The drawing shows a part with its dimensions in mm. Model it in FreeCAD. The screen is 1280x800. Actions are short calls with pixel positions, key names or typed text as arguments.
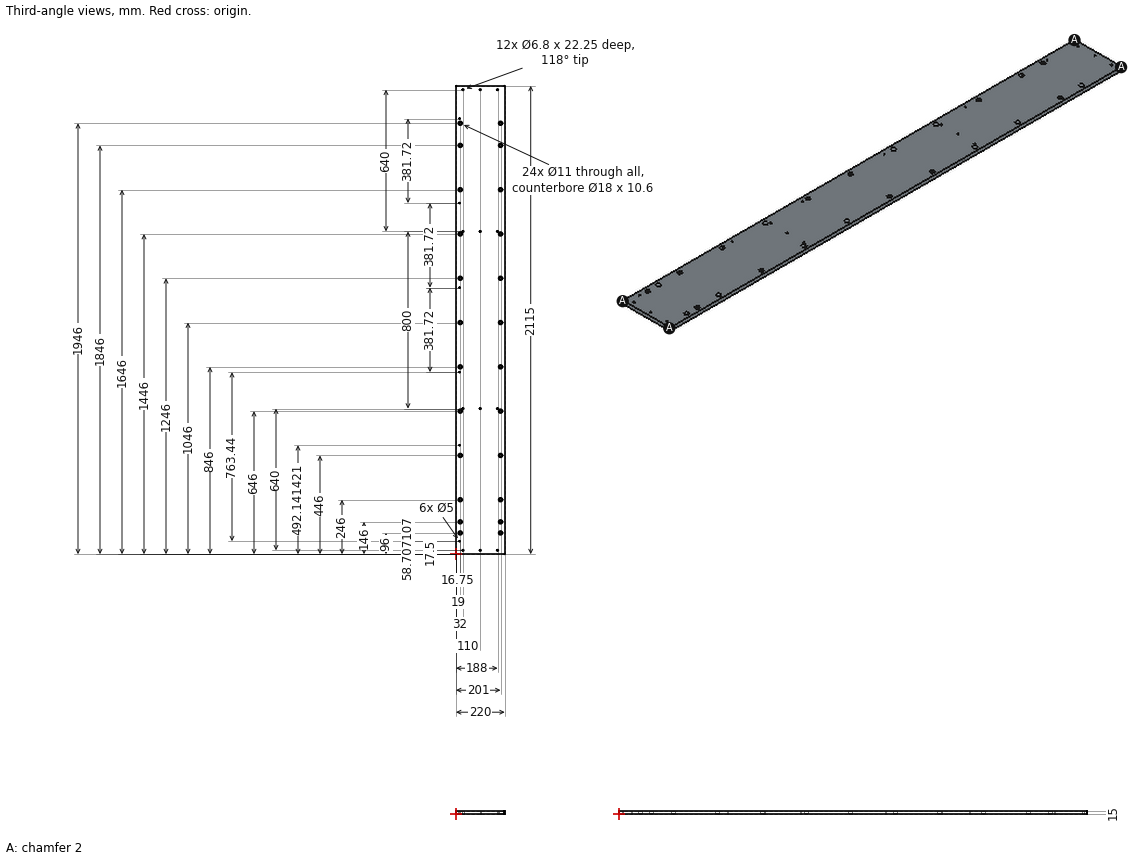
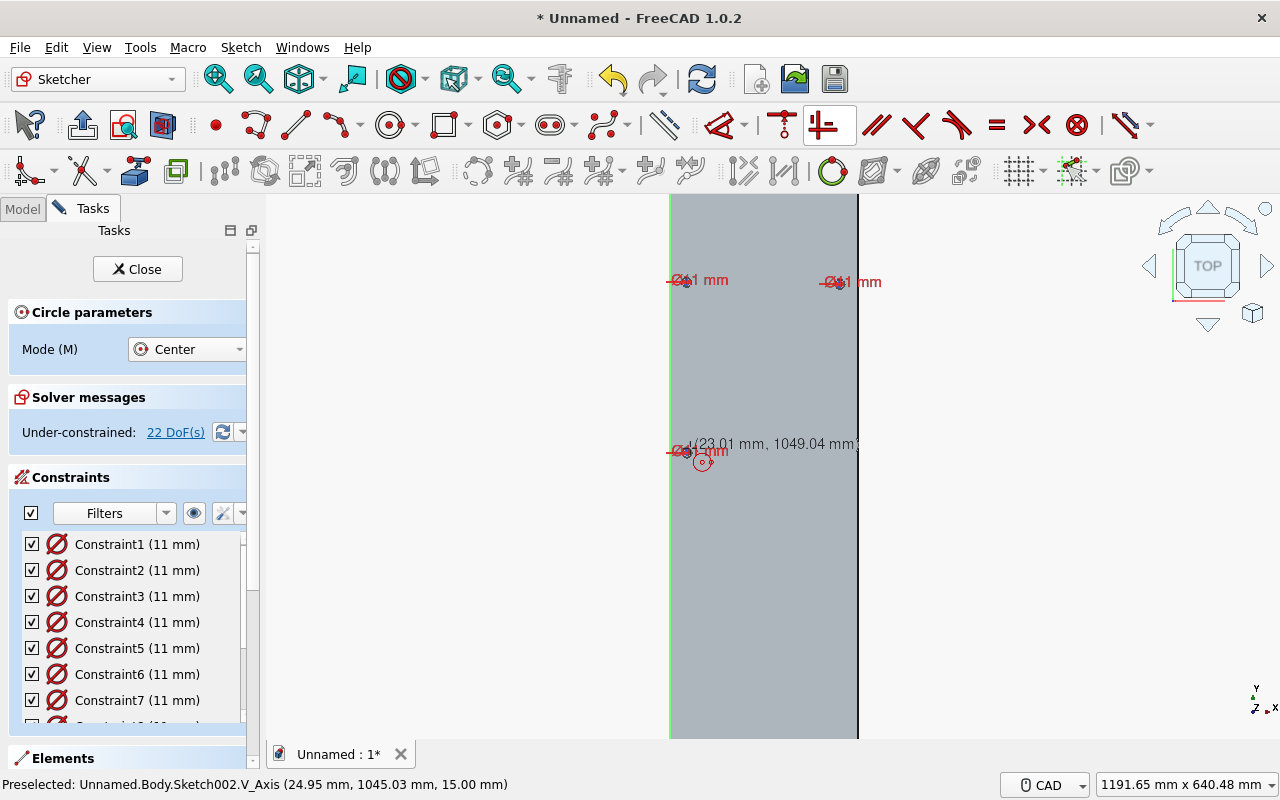
scroll(841, 452, up, 8)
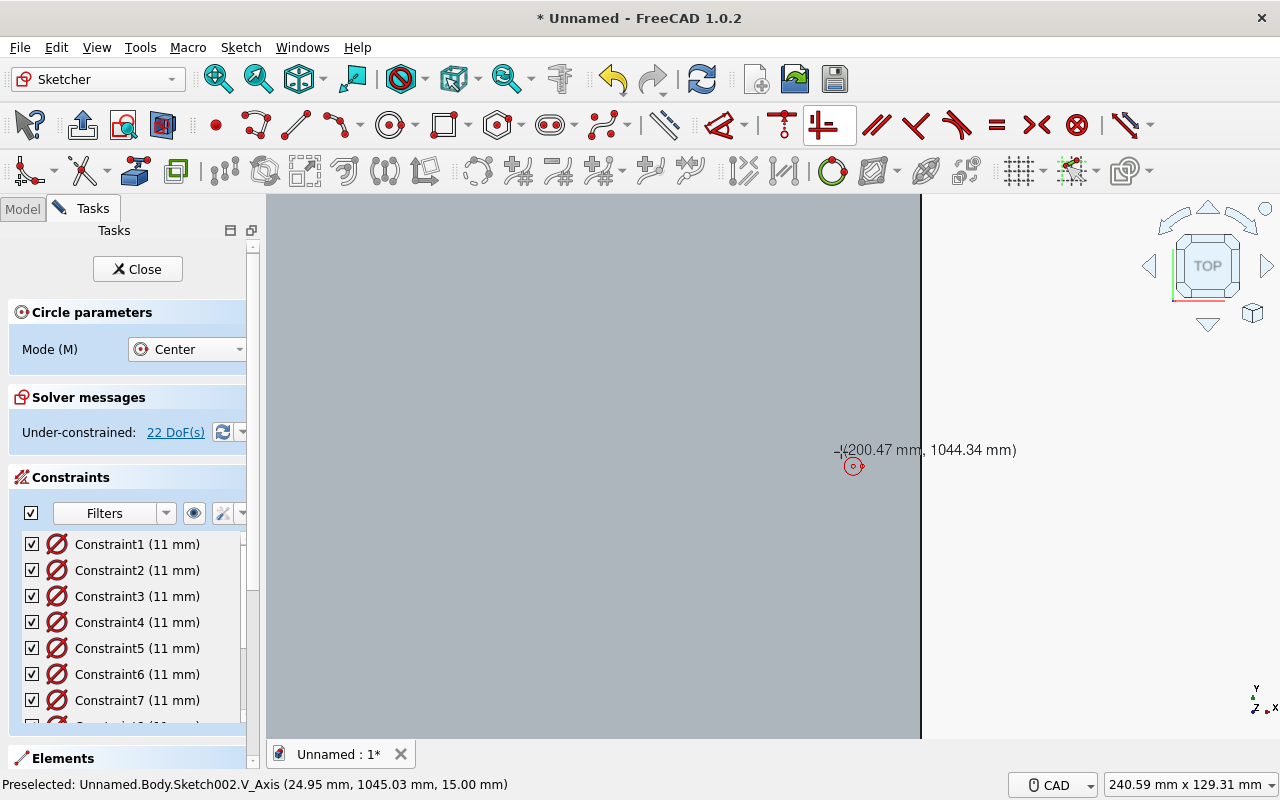
scroll(719, 452, down, 15)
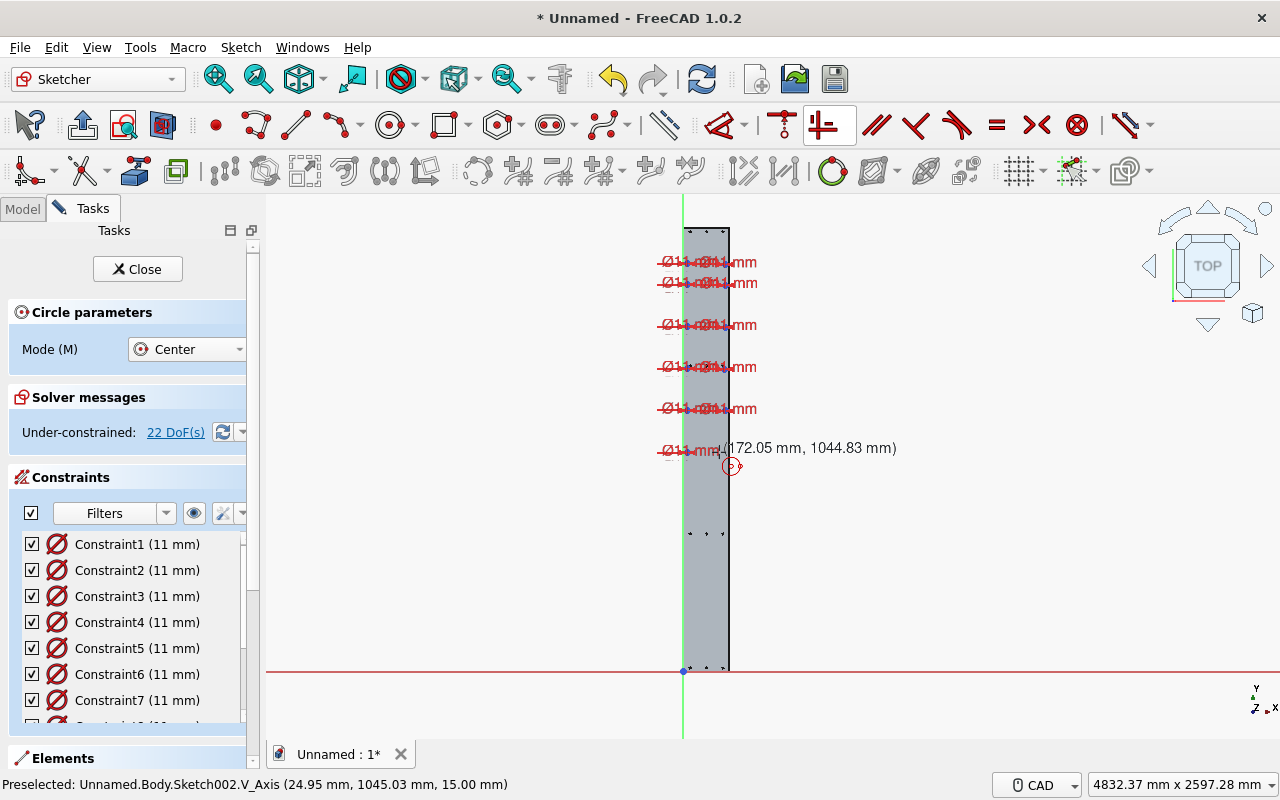
click(725, 452)
move(726, 451)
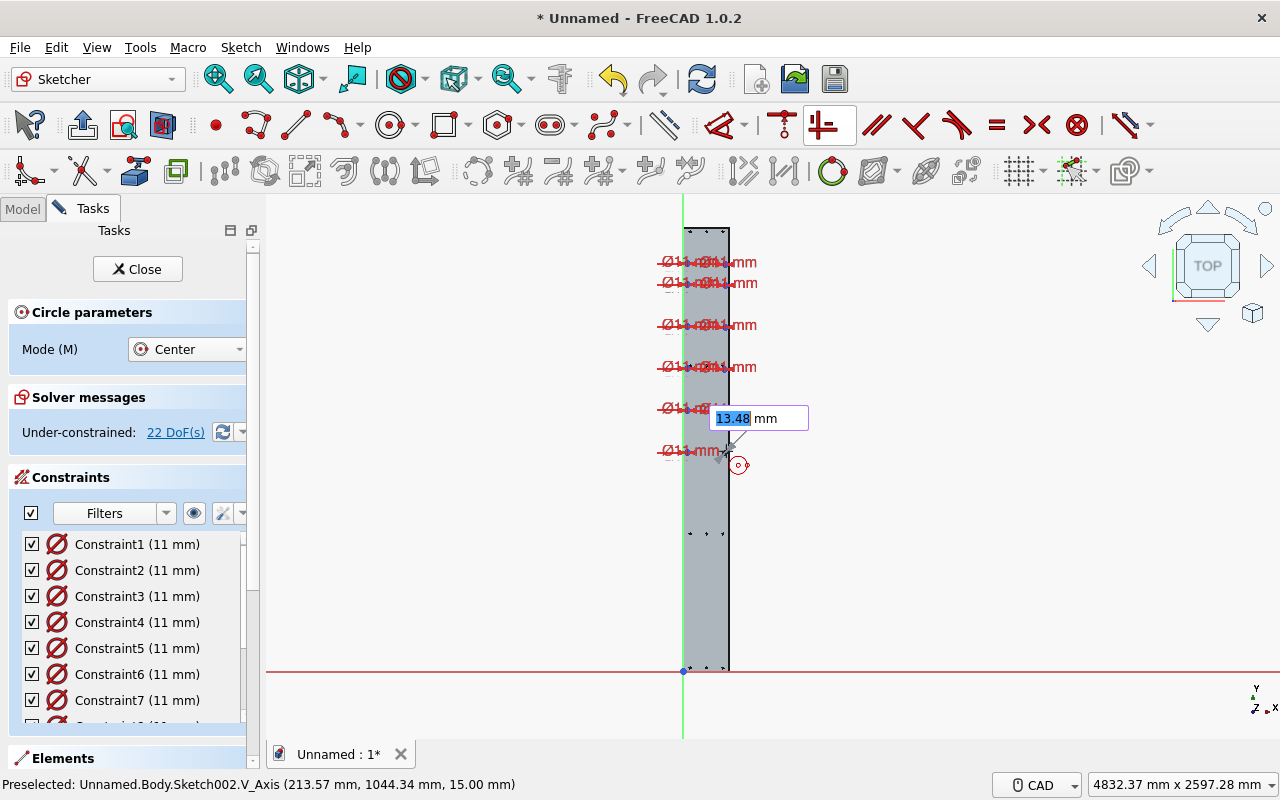
text(11)
key(Return)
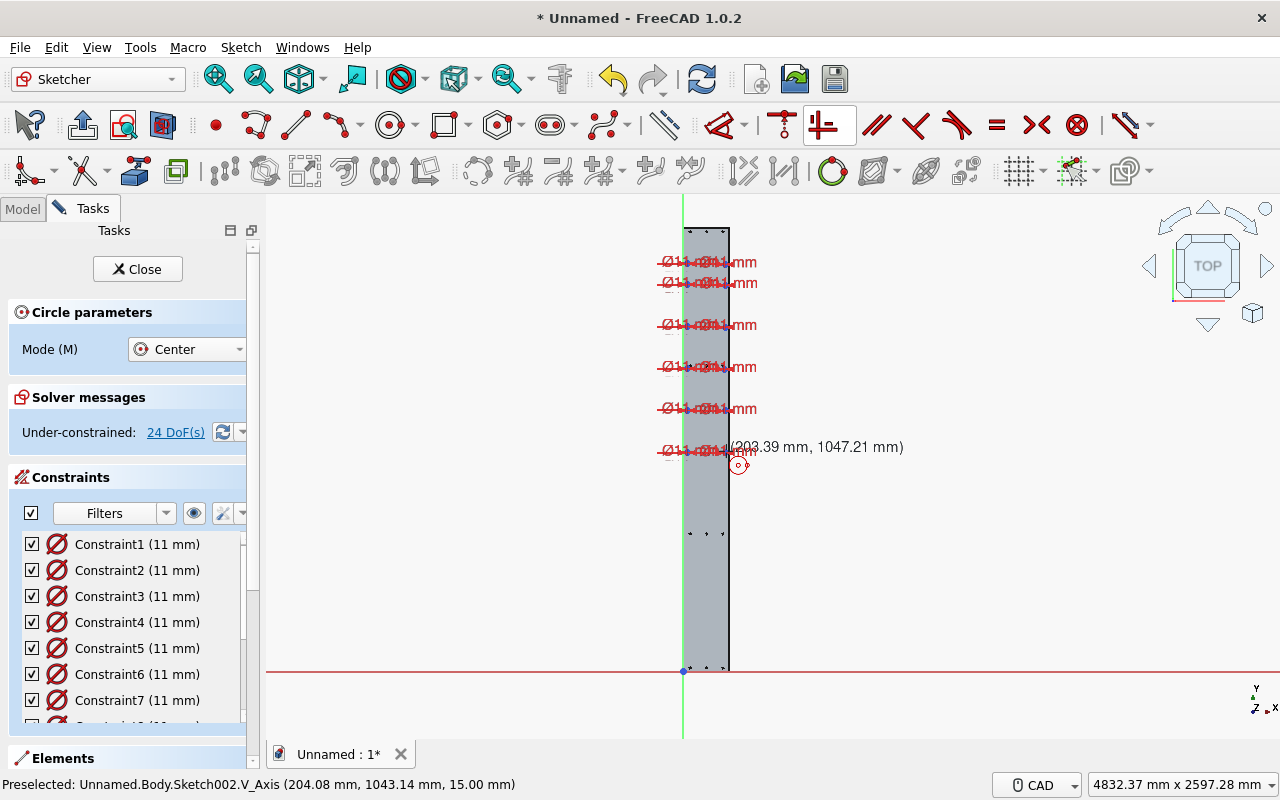
scroll(687, 494, up, 15)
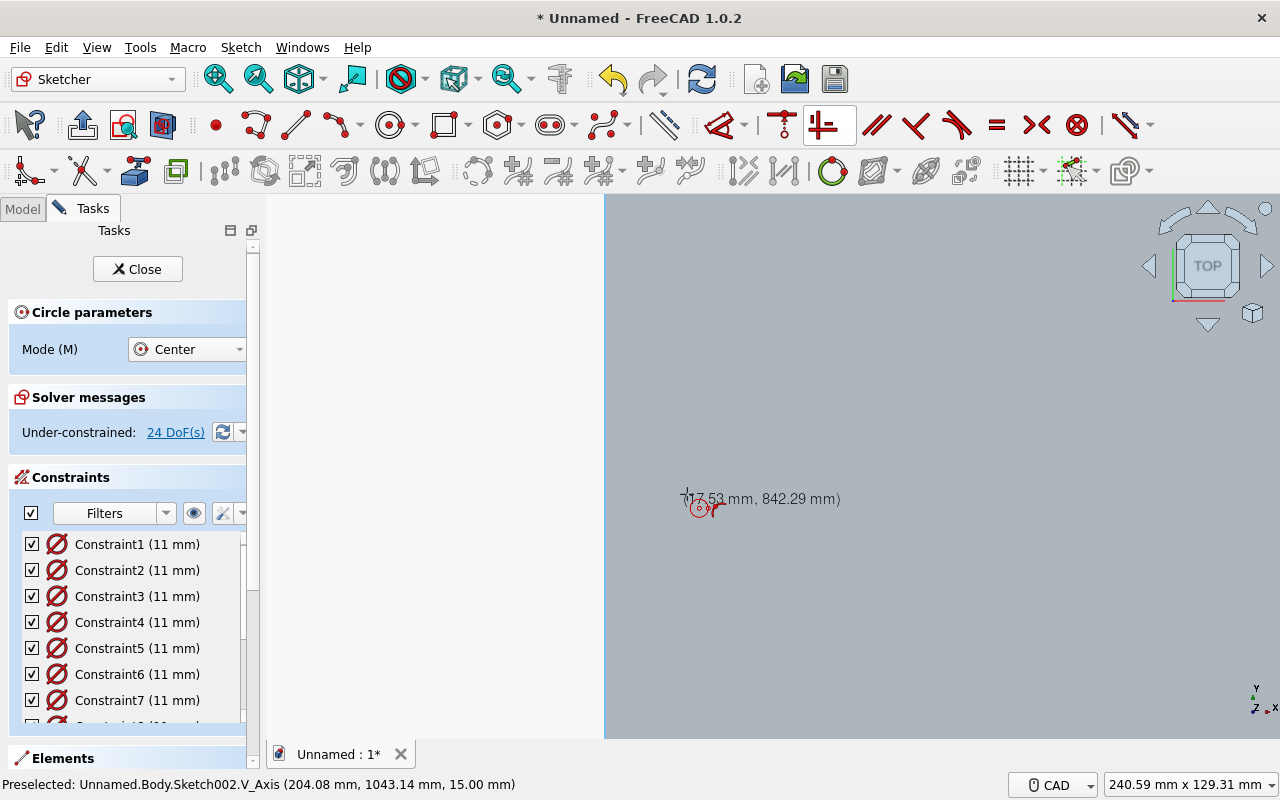
scroll(687, 494, down, 15)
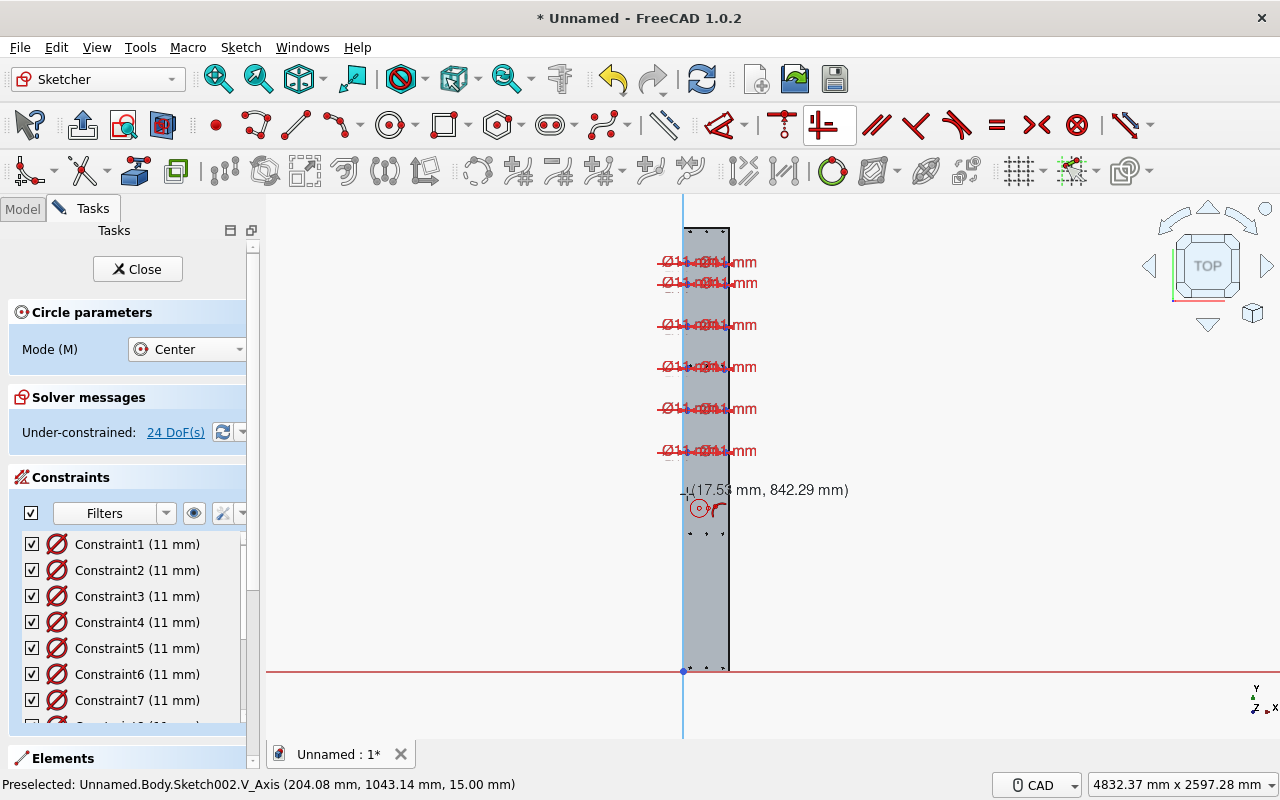
scroll(687, 494, up, 7)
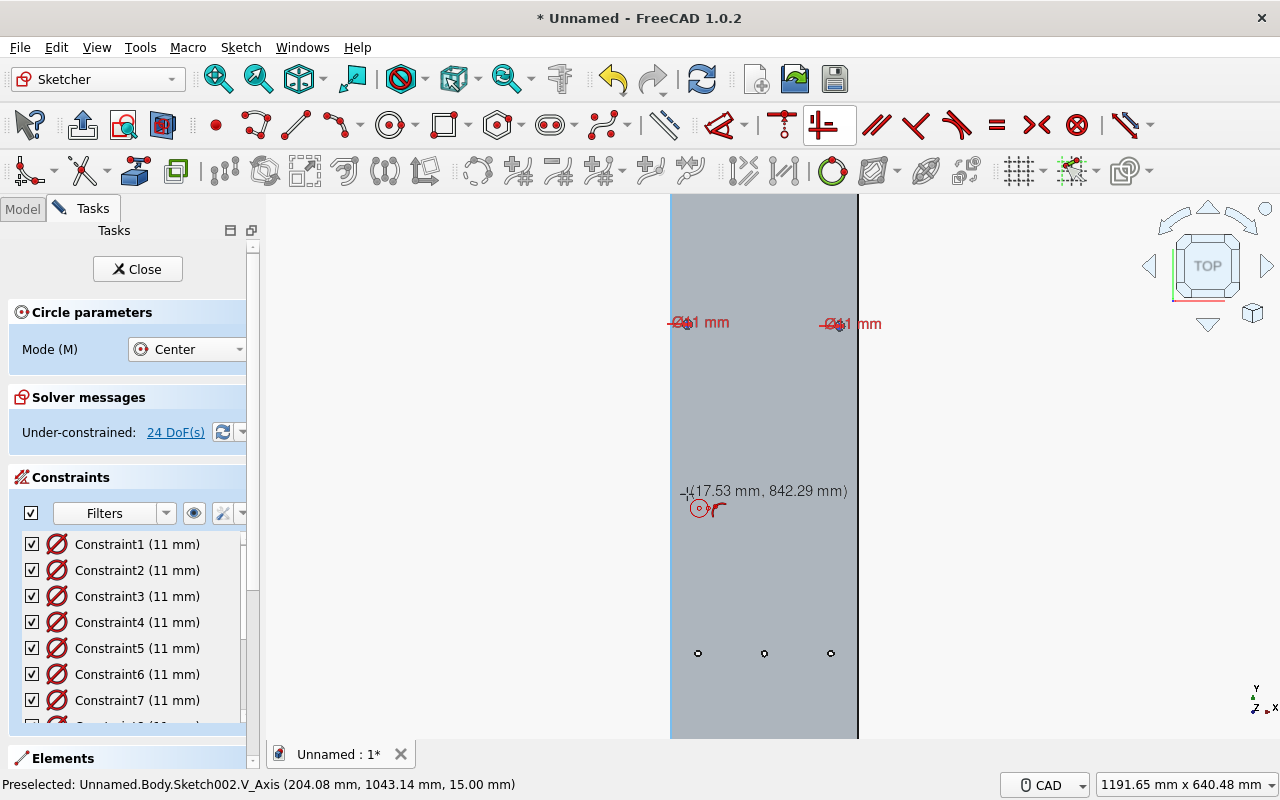
click(687, 493)
move(690, 490)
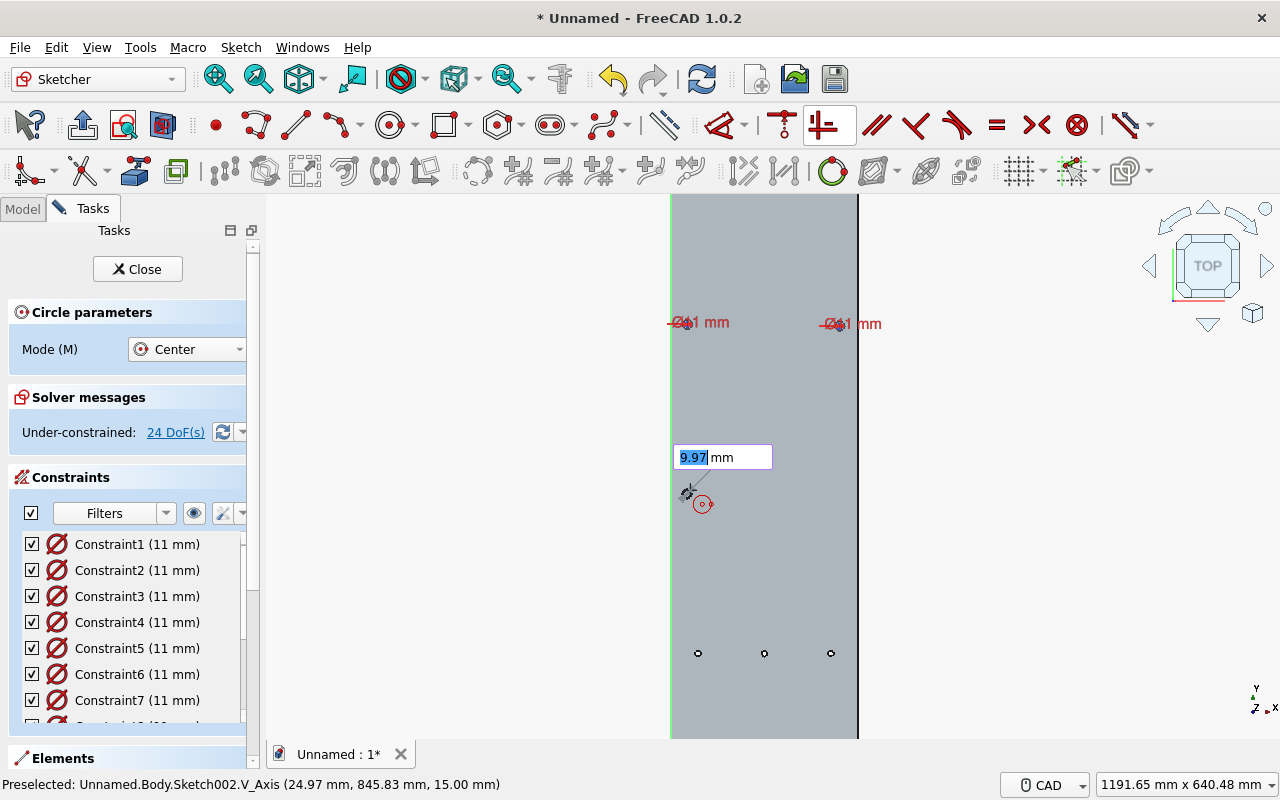
text(11)
key(Return)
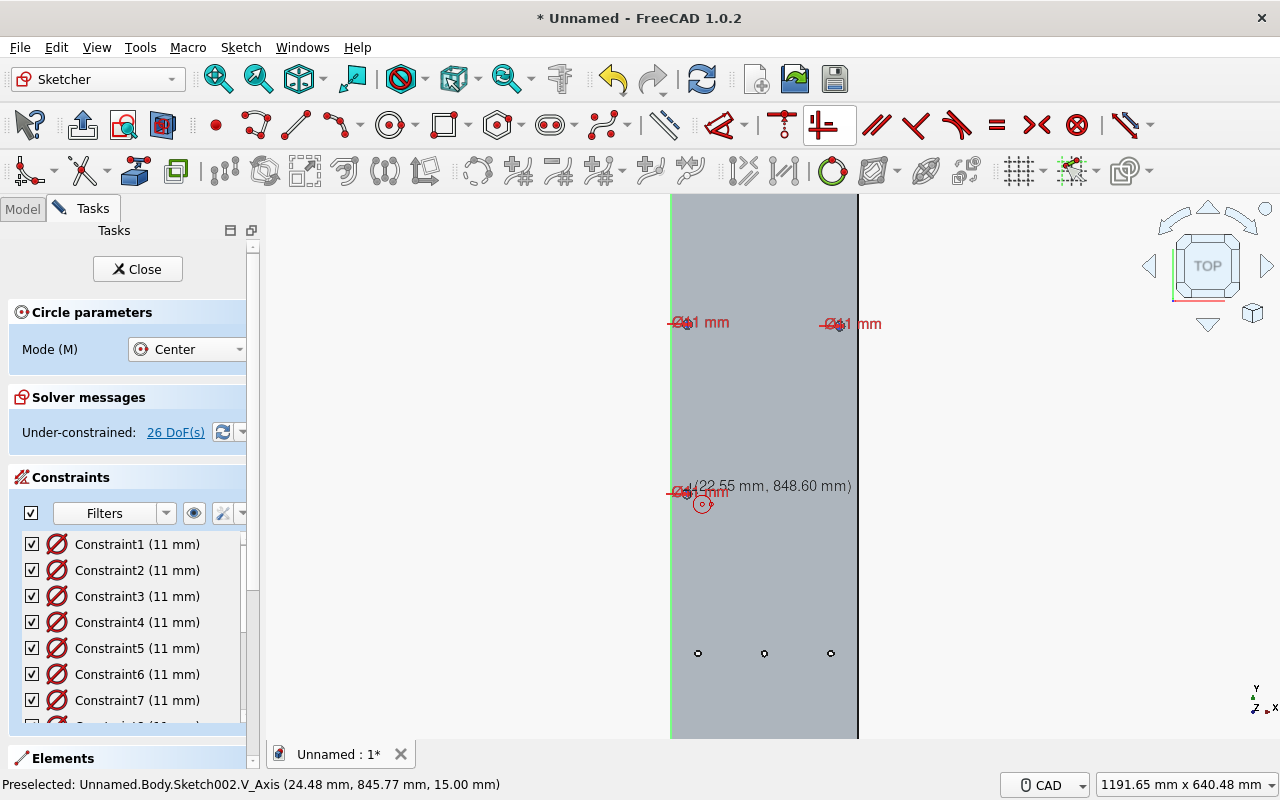
scroll(842, 493, up, 8)